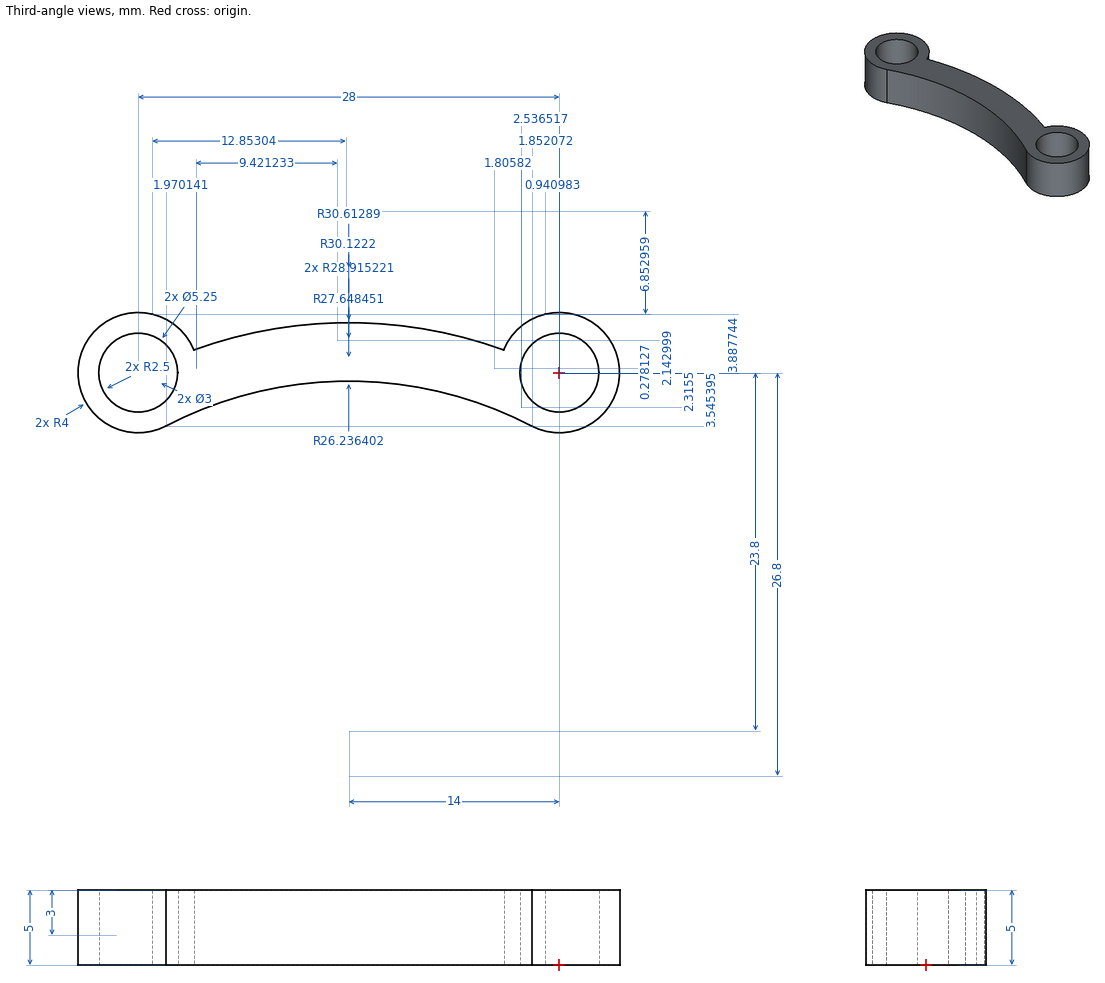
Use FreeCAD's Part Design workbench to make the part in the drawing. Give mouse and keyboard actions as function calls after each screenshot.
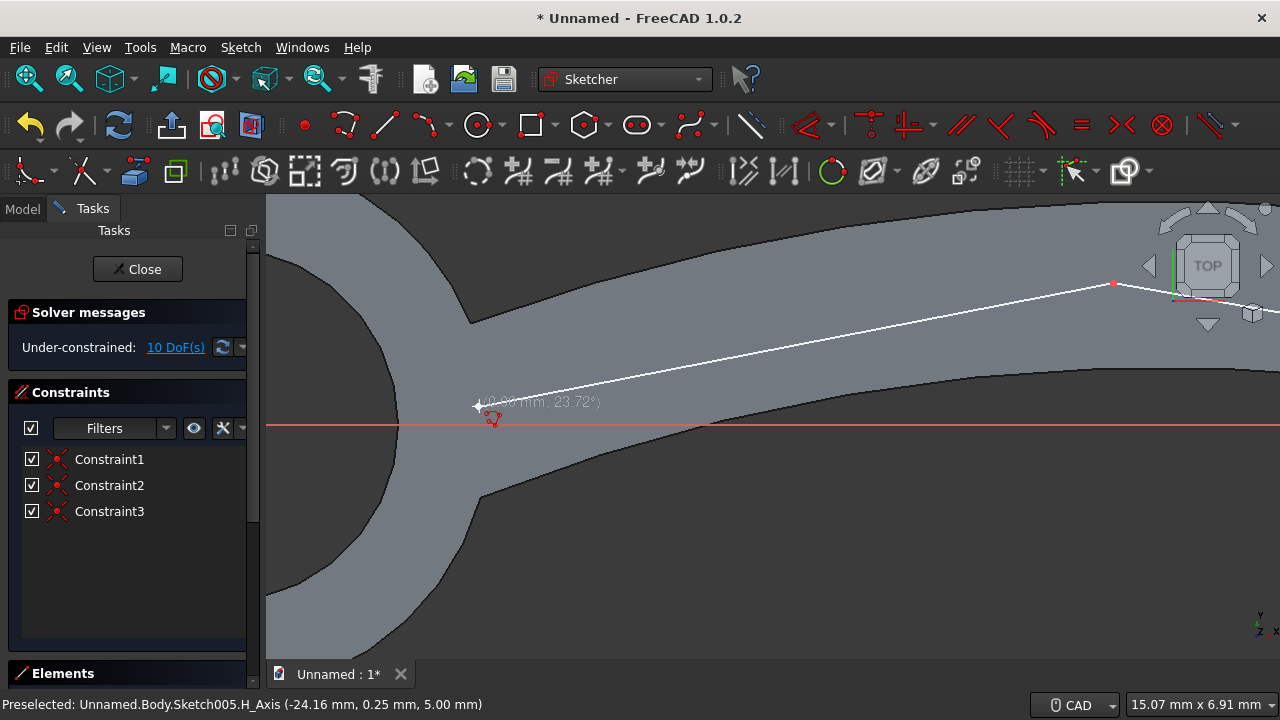
scroll(480, 407, down, 6)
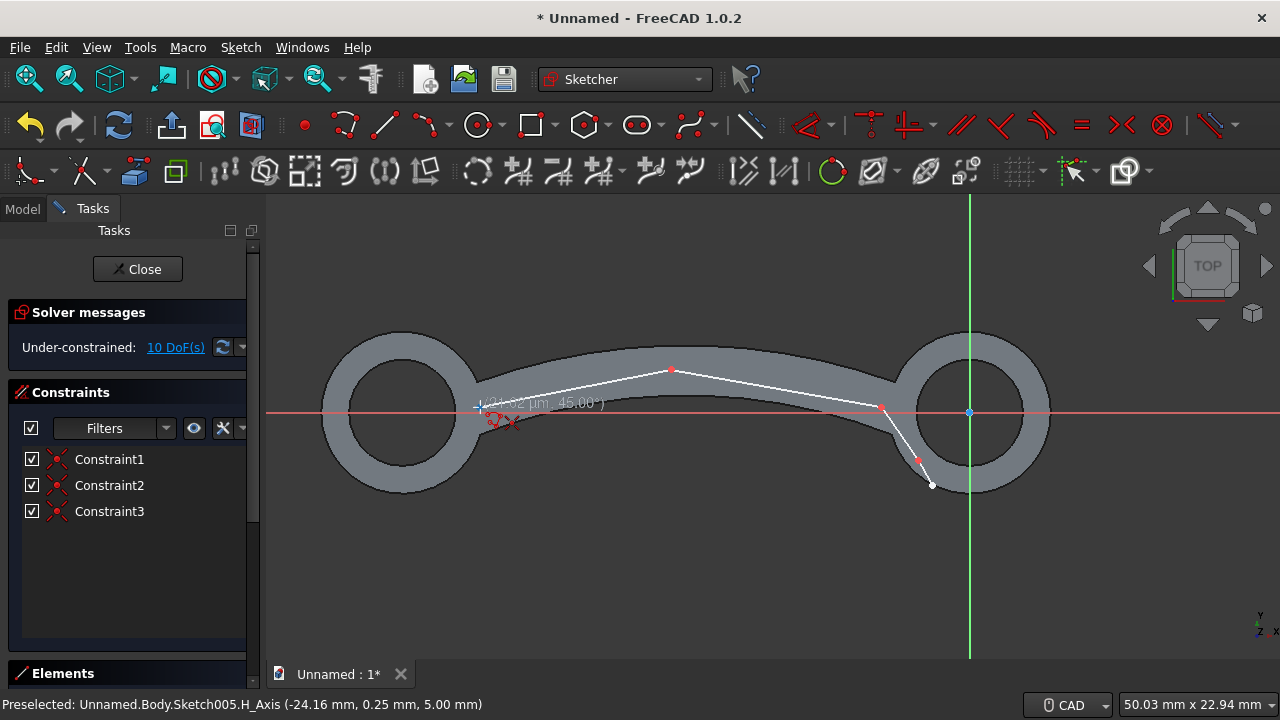
click(440, 485)
right_click(440, 485)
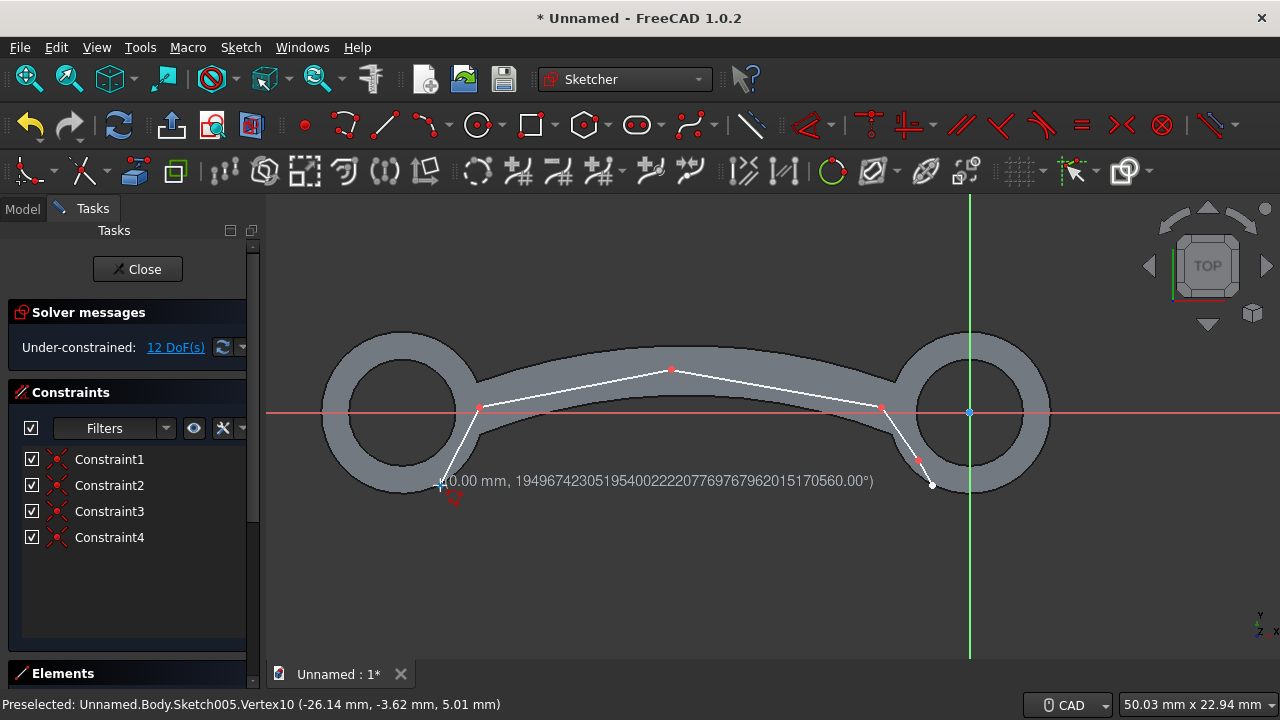
click(426, 126)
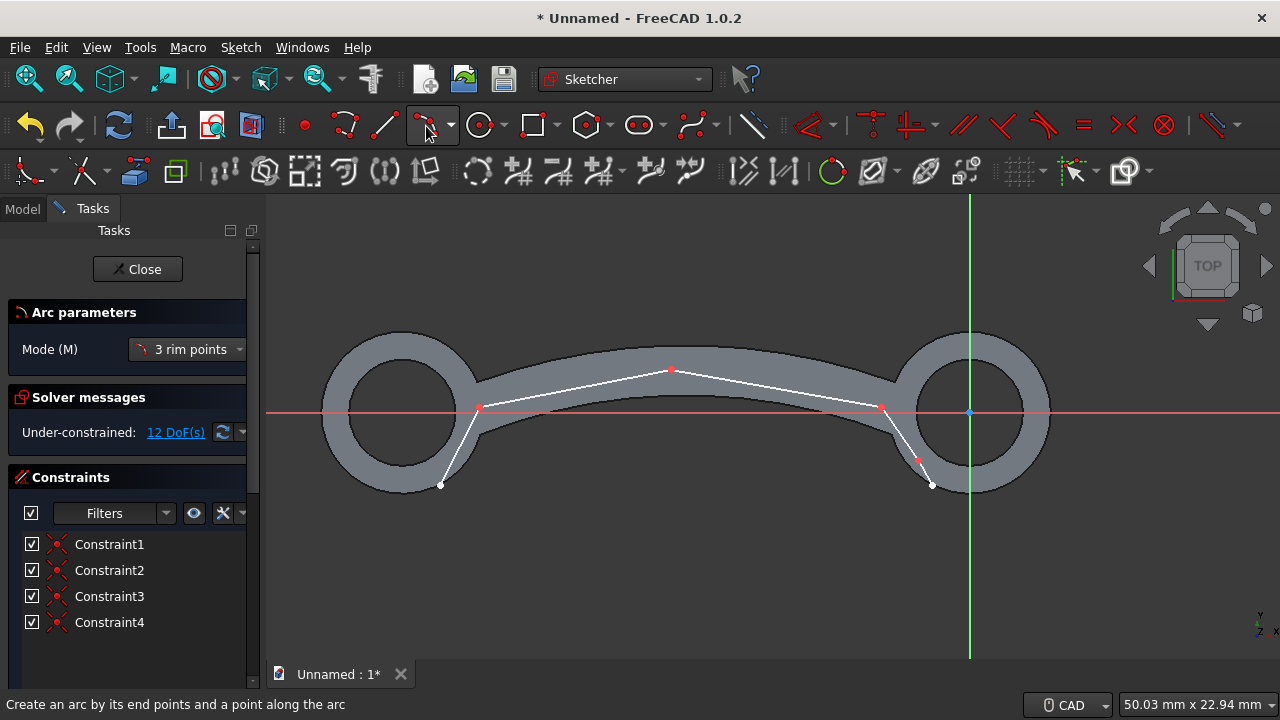
click(440, 486)
click(933, 486)
click(788, 434)
key(Escape)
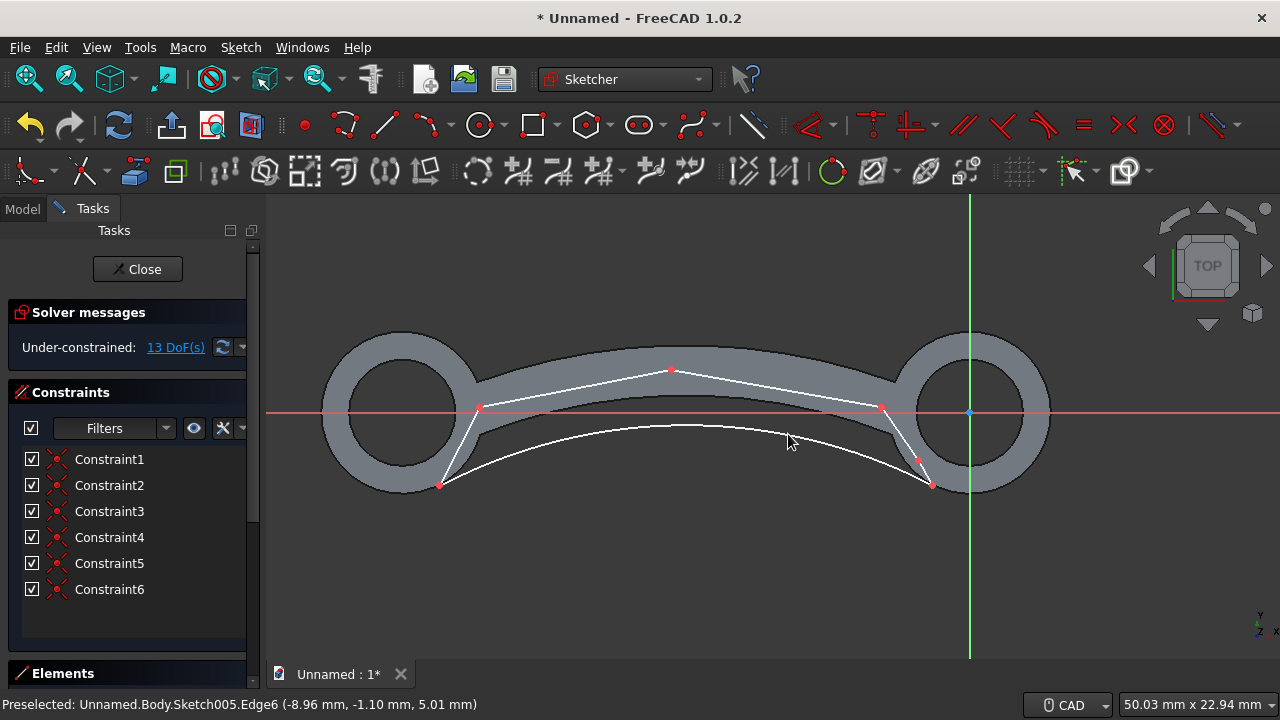
click(808, 126)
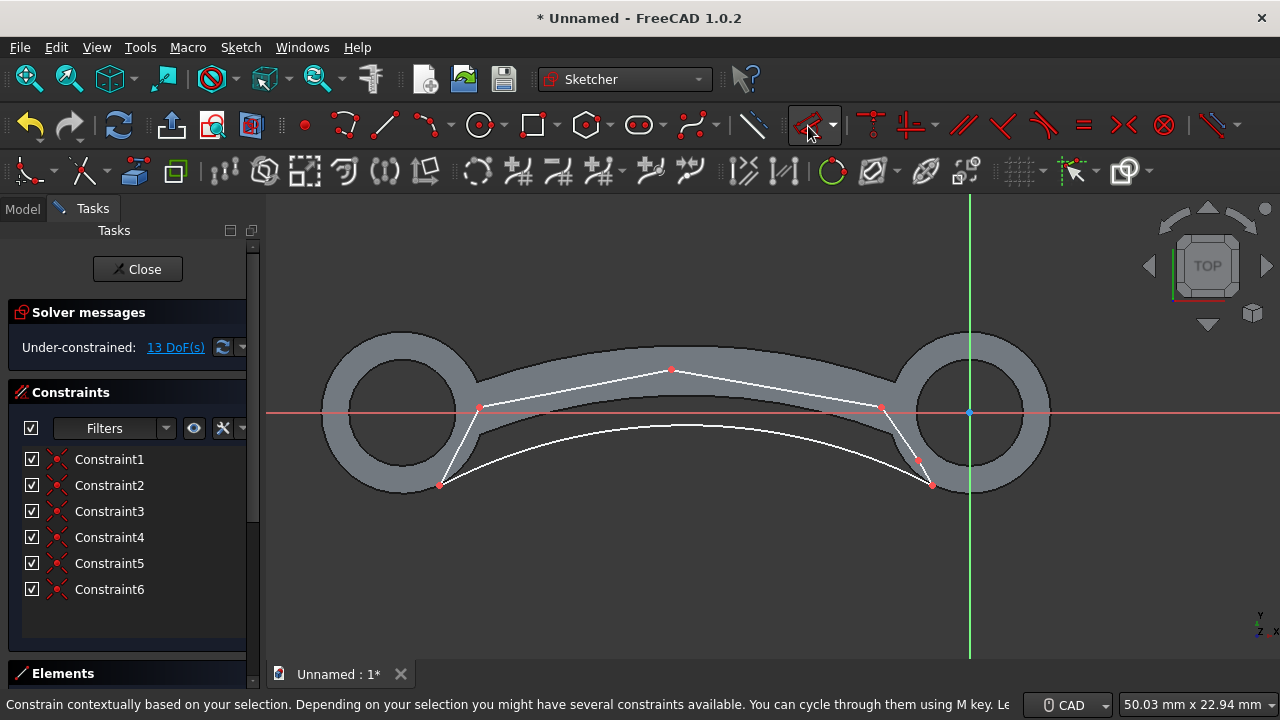
click(788, 435)
click(1046, 523)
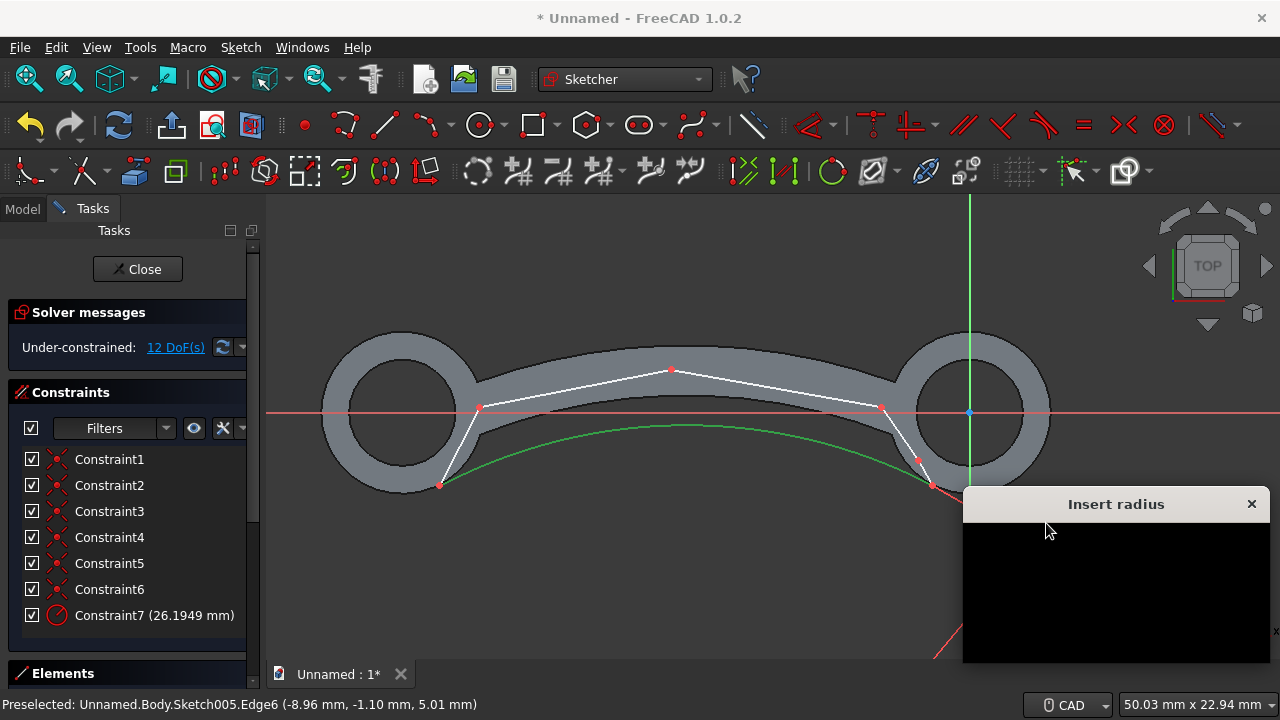
text(26.236402)
key(Return)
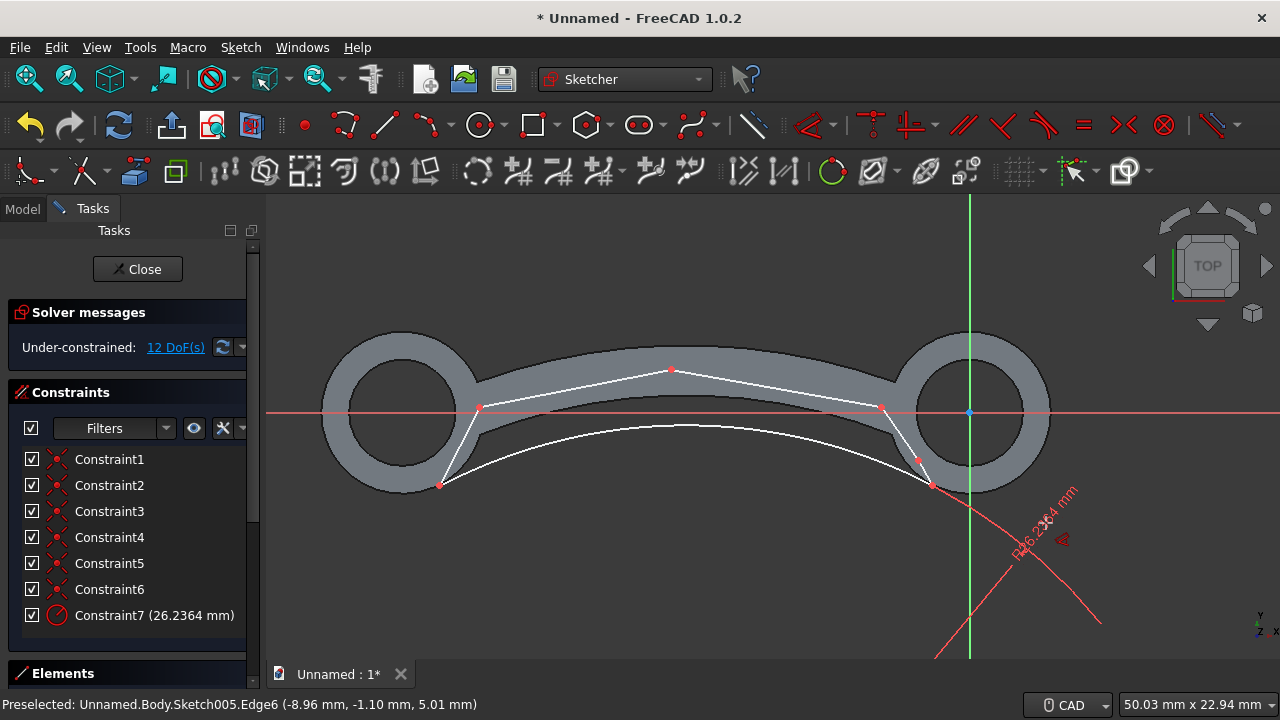
scroll(704, 233, down, 4)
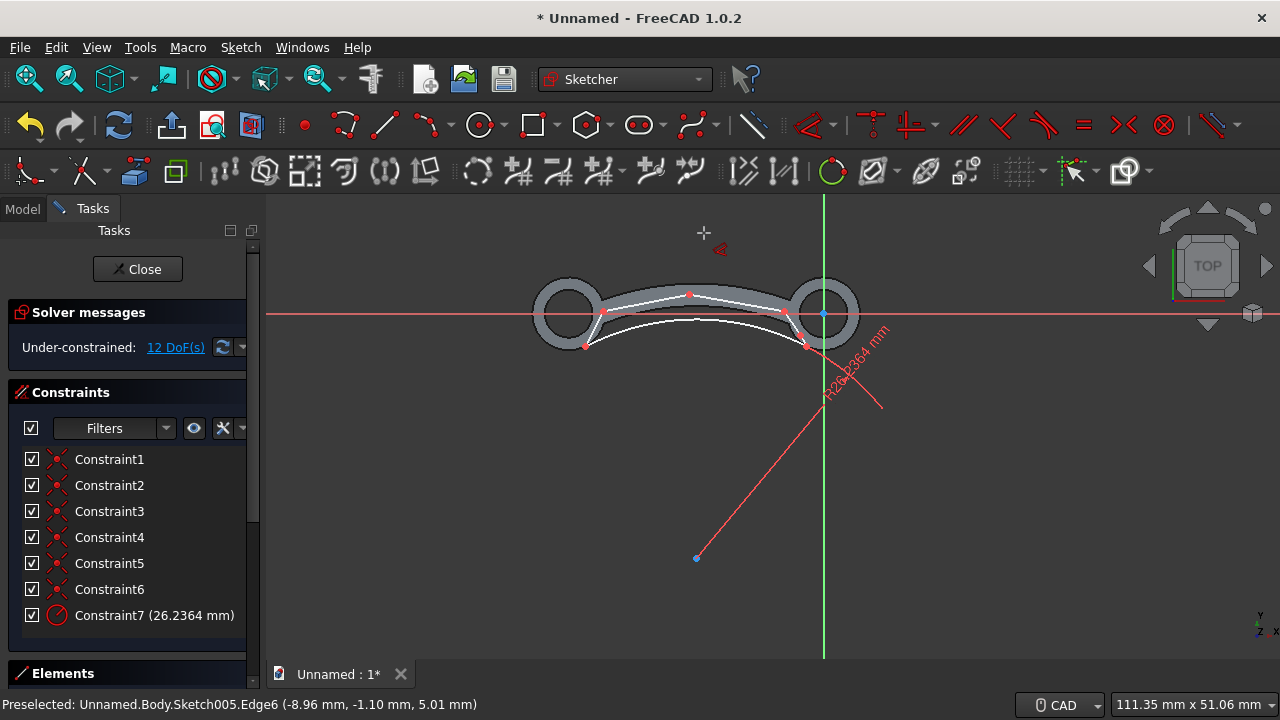
click(696, 558)
click(760, 592)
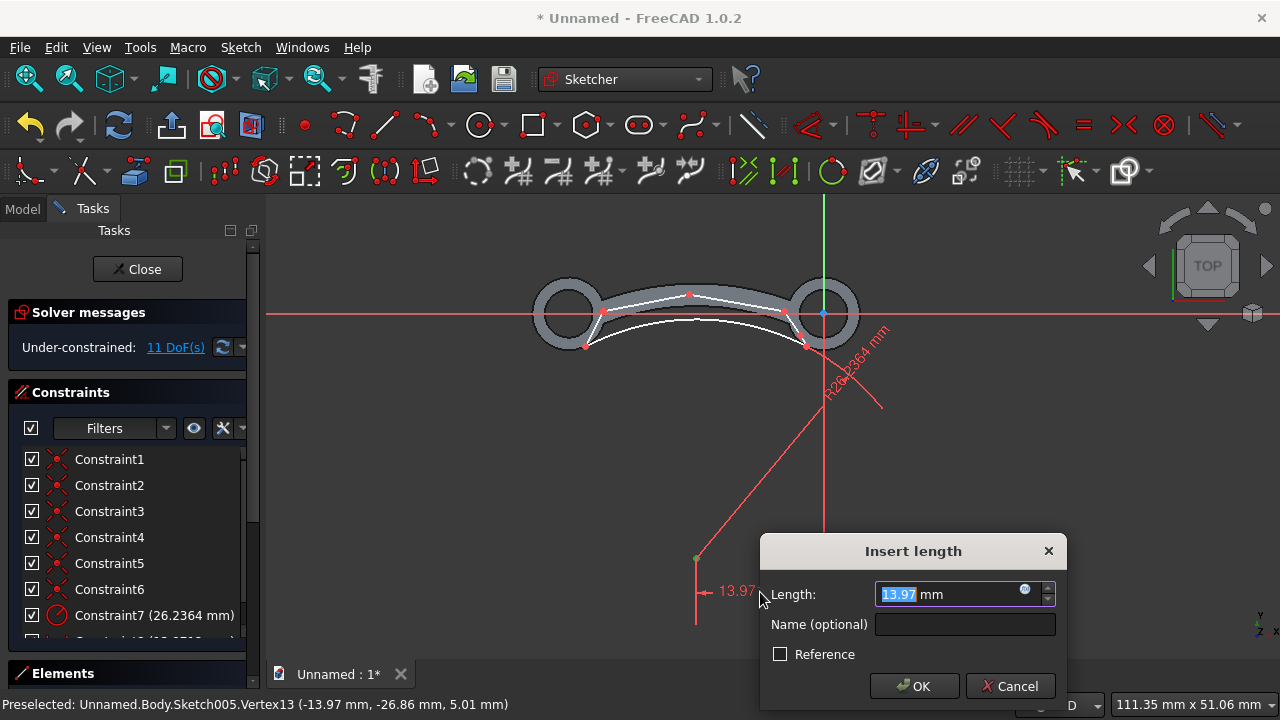
text(14)
key(Return)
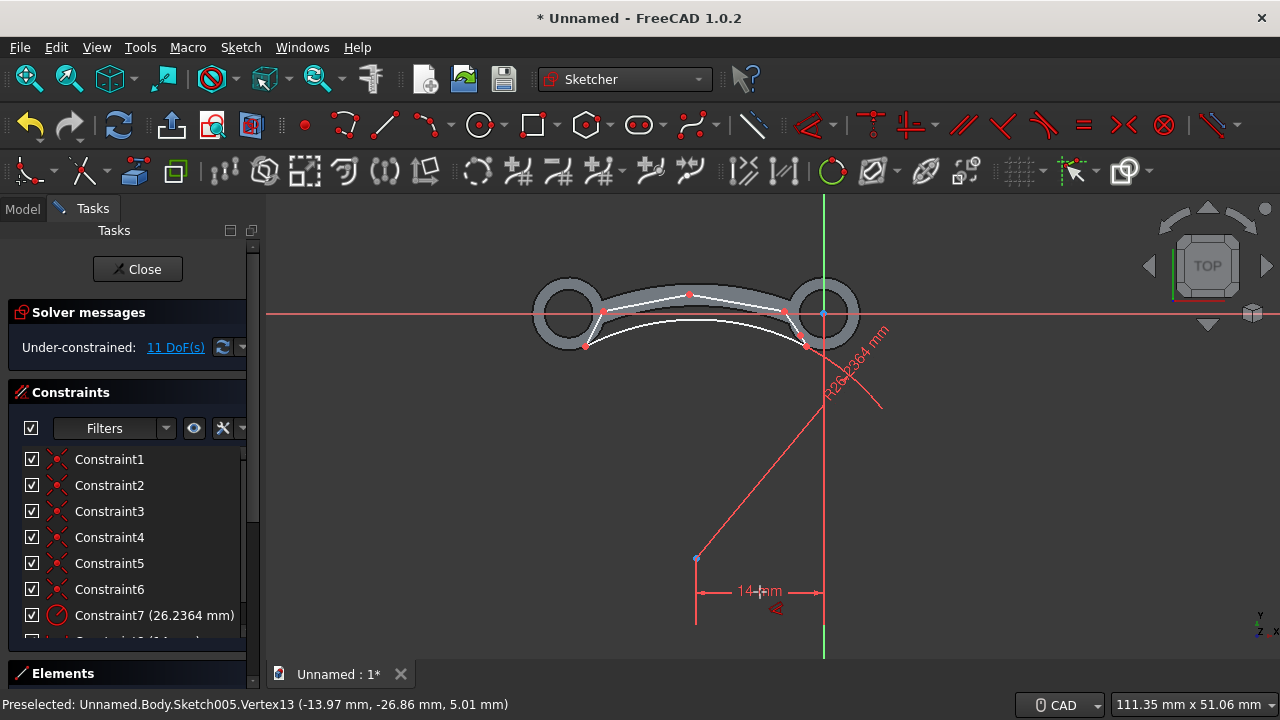
click(696, 559)
click(858, 436)